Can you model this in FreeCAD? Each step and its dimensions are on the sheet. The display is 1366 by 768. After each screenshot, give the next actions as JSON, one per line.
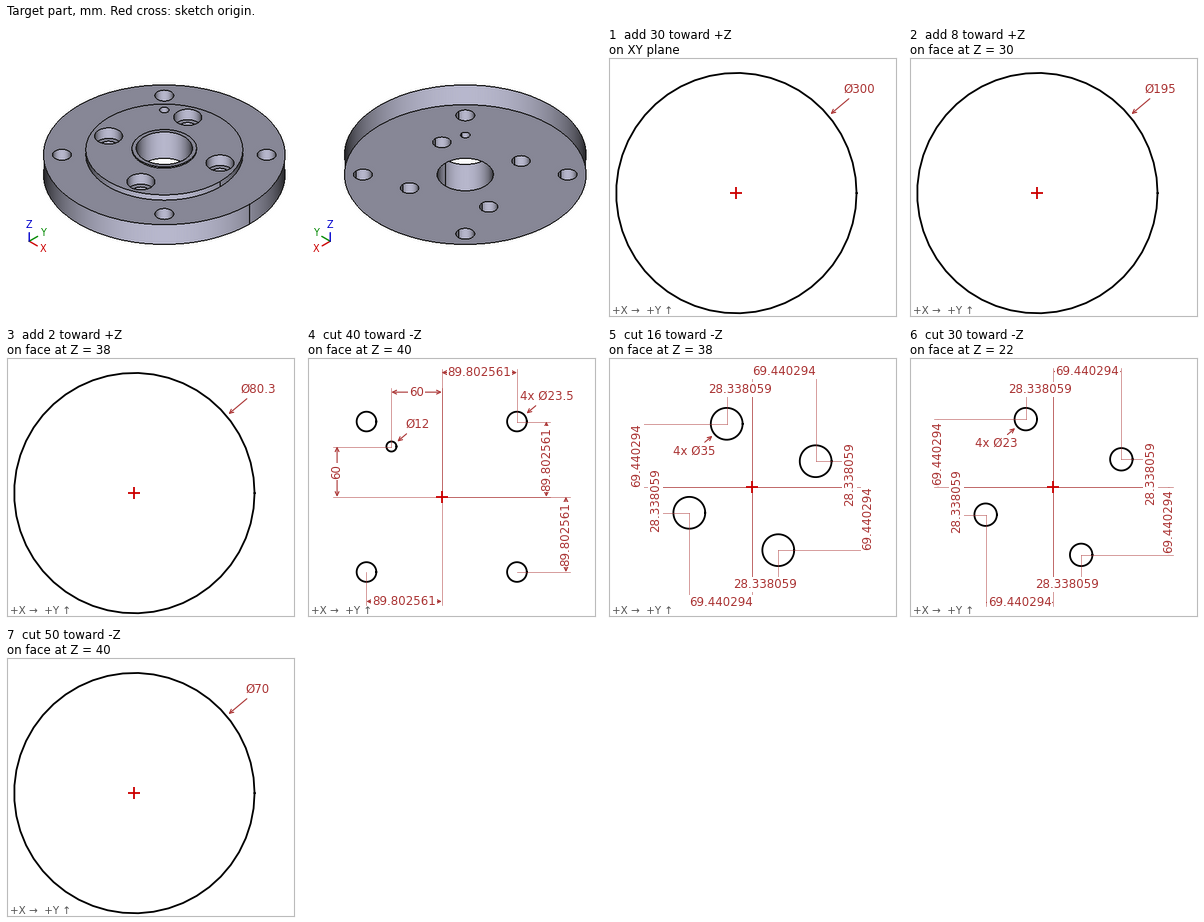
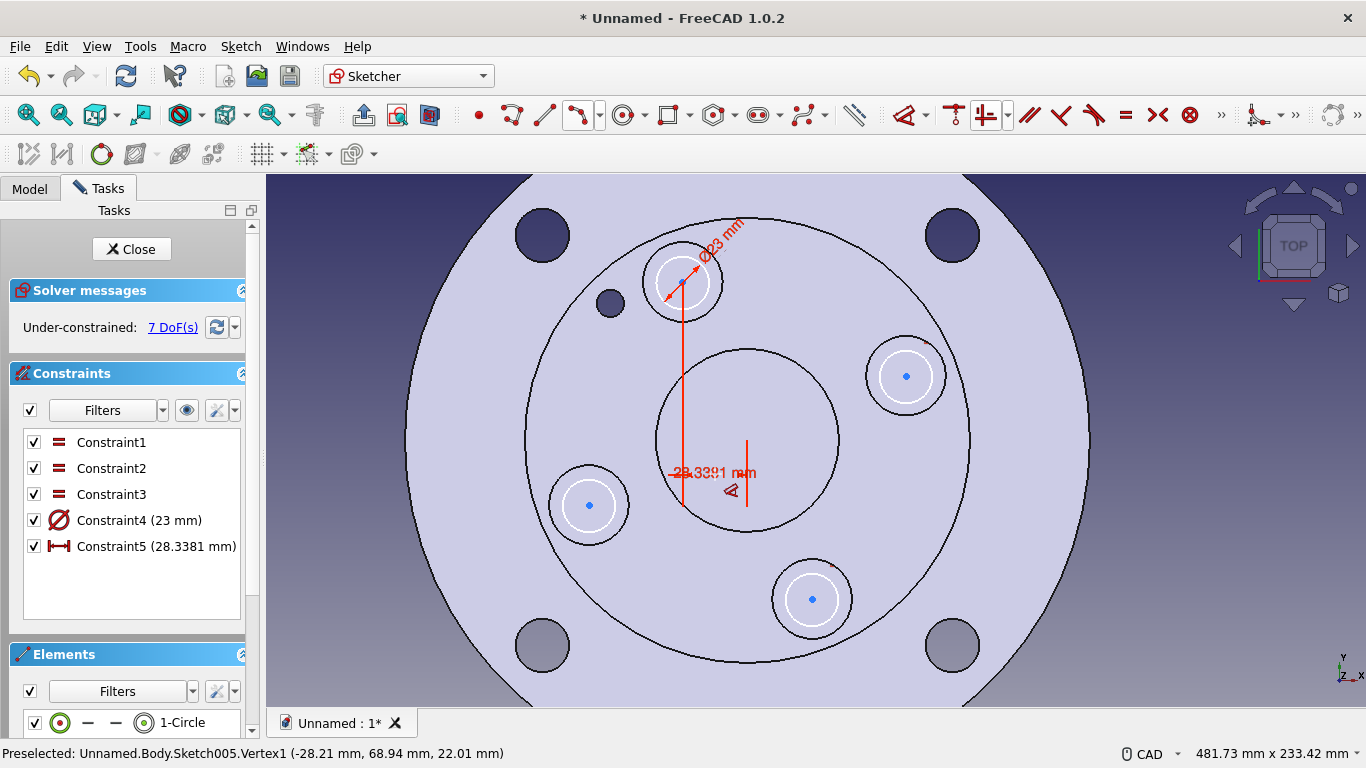
{"action": "left_click", "coordinate": [683, 283]}
{"action": "left_click", "coordinate": [649, 362]}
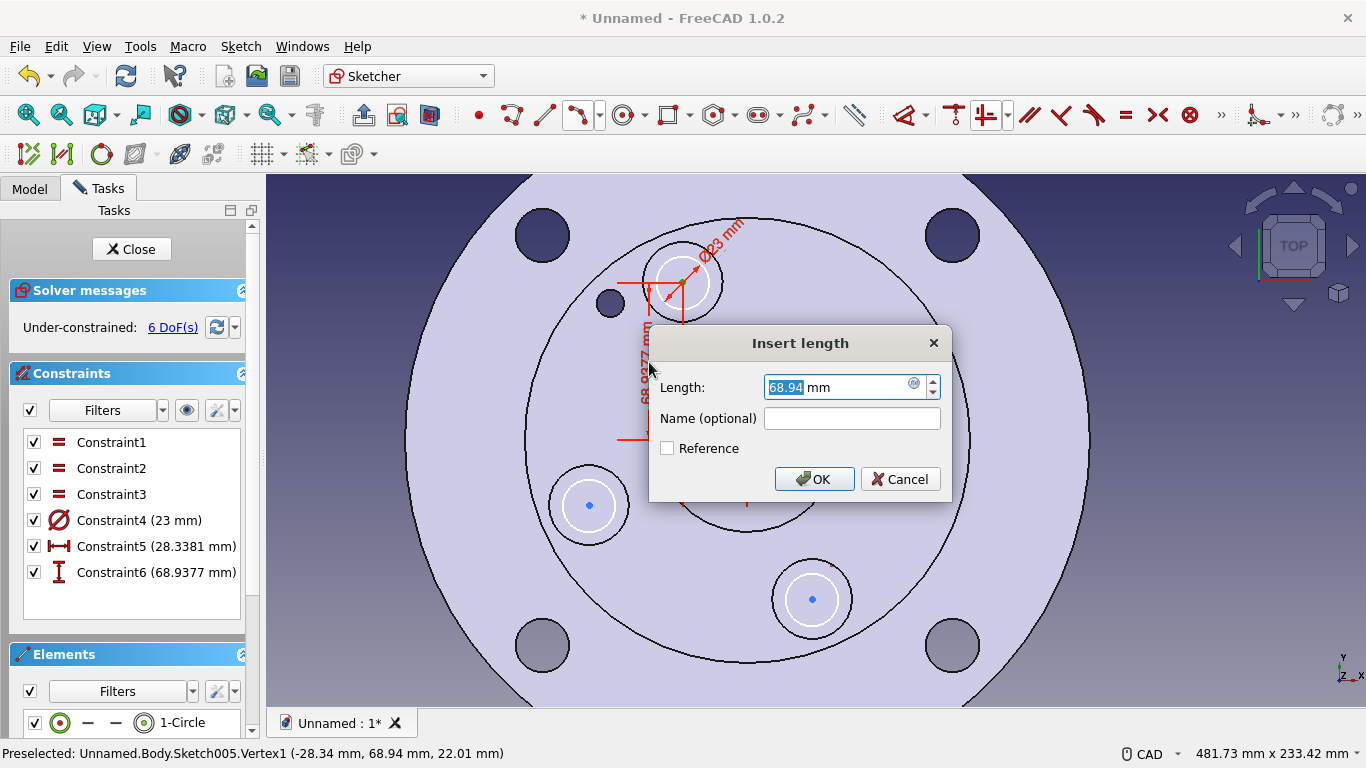
{"action": "type", "text": "69.440294"}
{"action": "key", "text": "Return"}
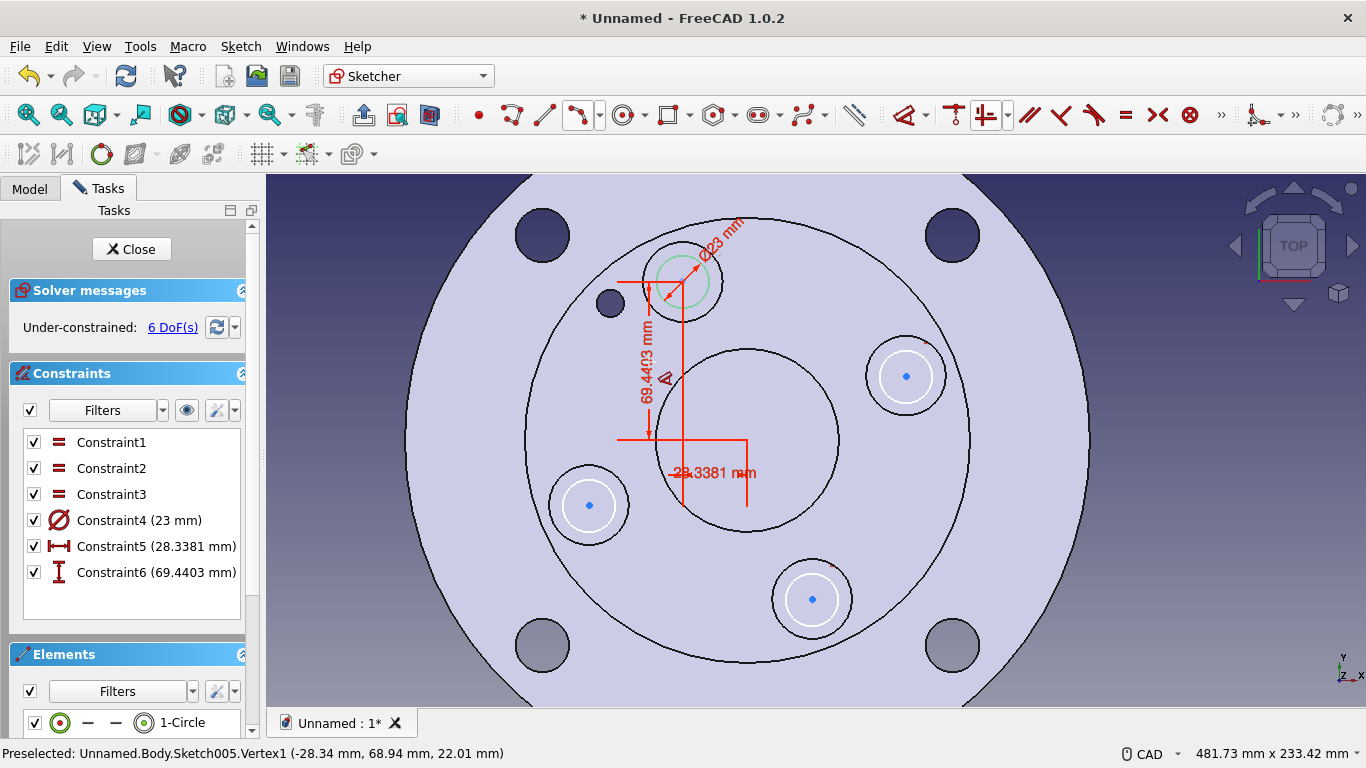
{"action": "left_click", "coordinate": [906, 377]}
{"action": "left_click", "coordinate": [827, 343]}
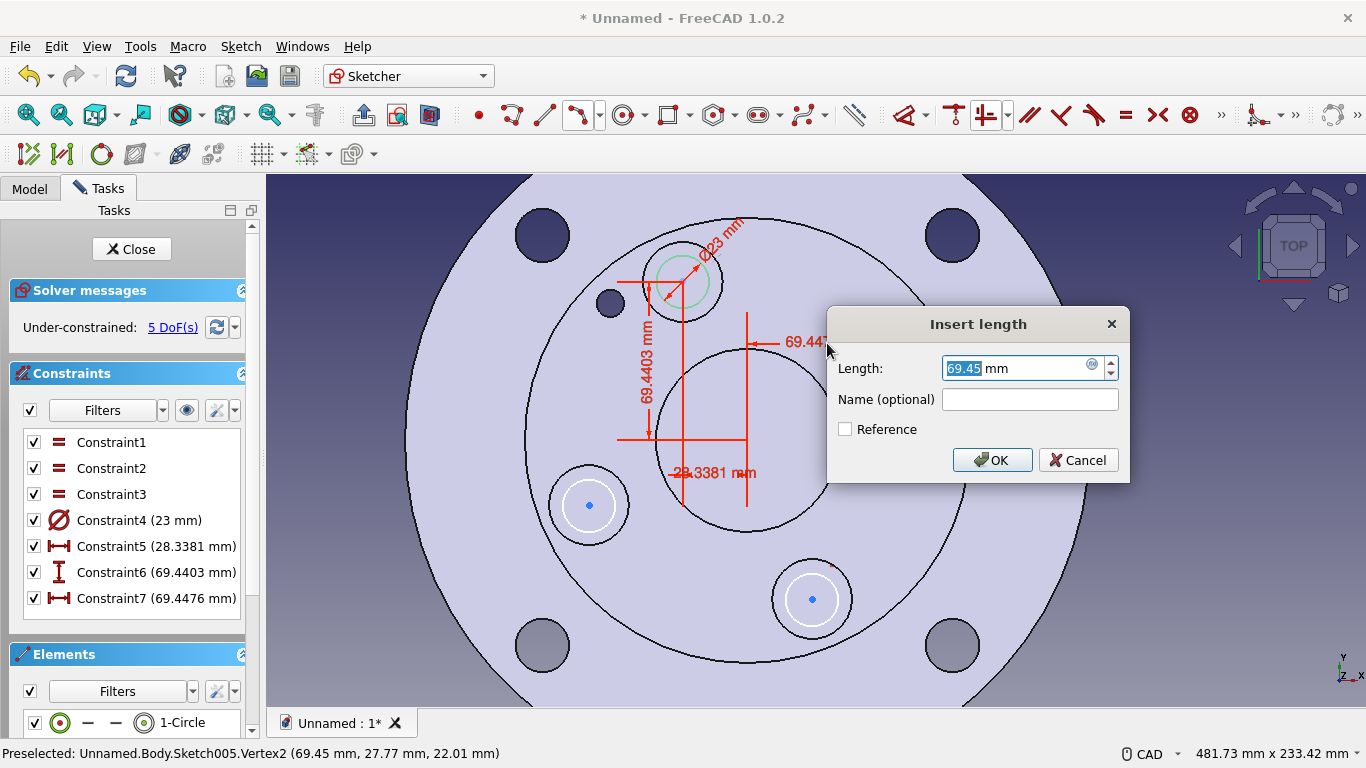
{"action": "type", "text": "69.440294"}
{"action": "key", "text": "Return"}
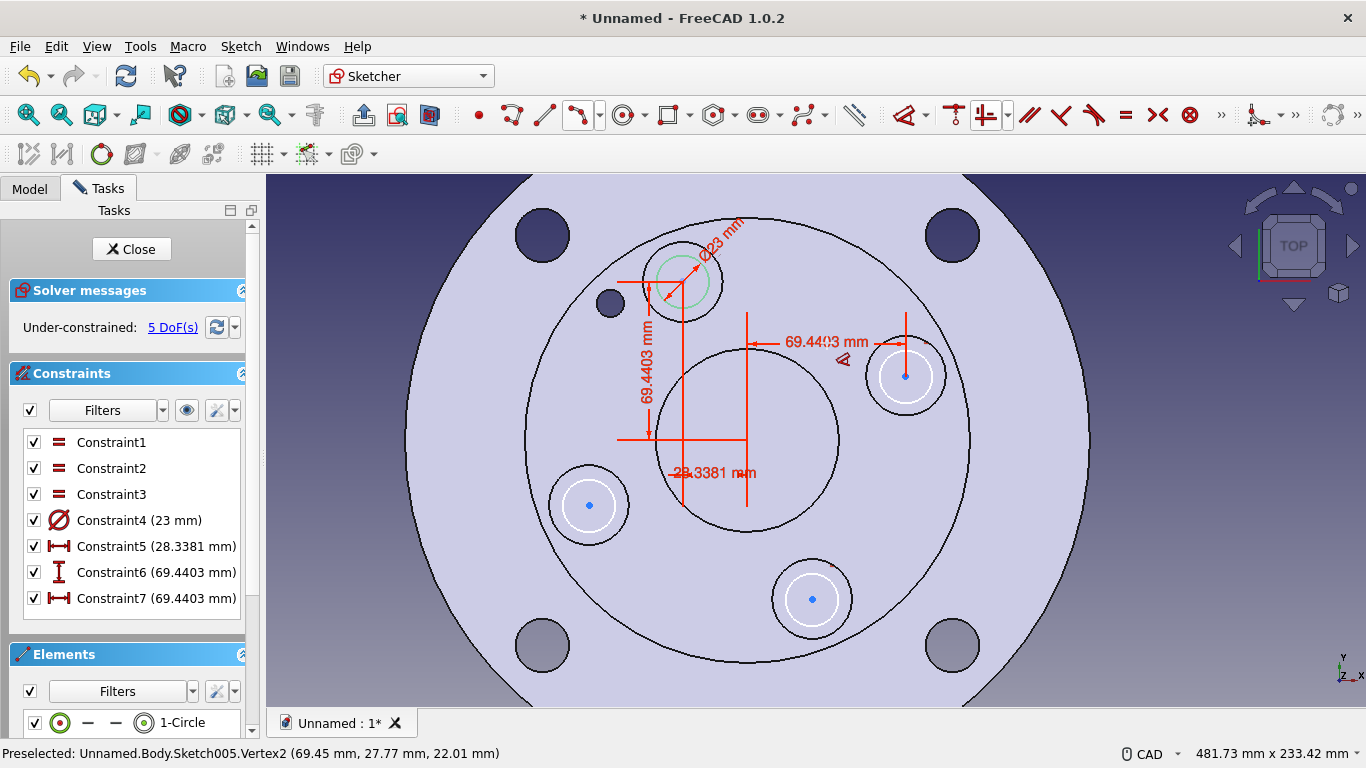
{"action": "left_click", "coordinate": [906, 377]}
{"action": "left_click", "coordinate": [940, 409]}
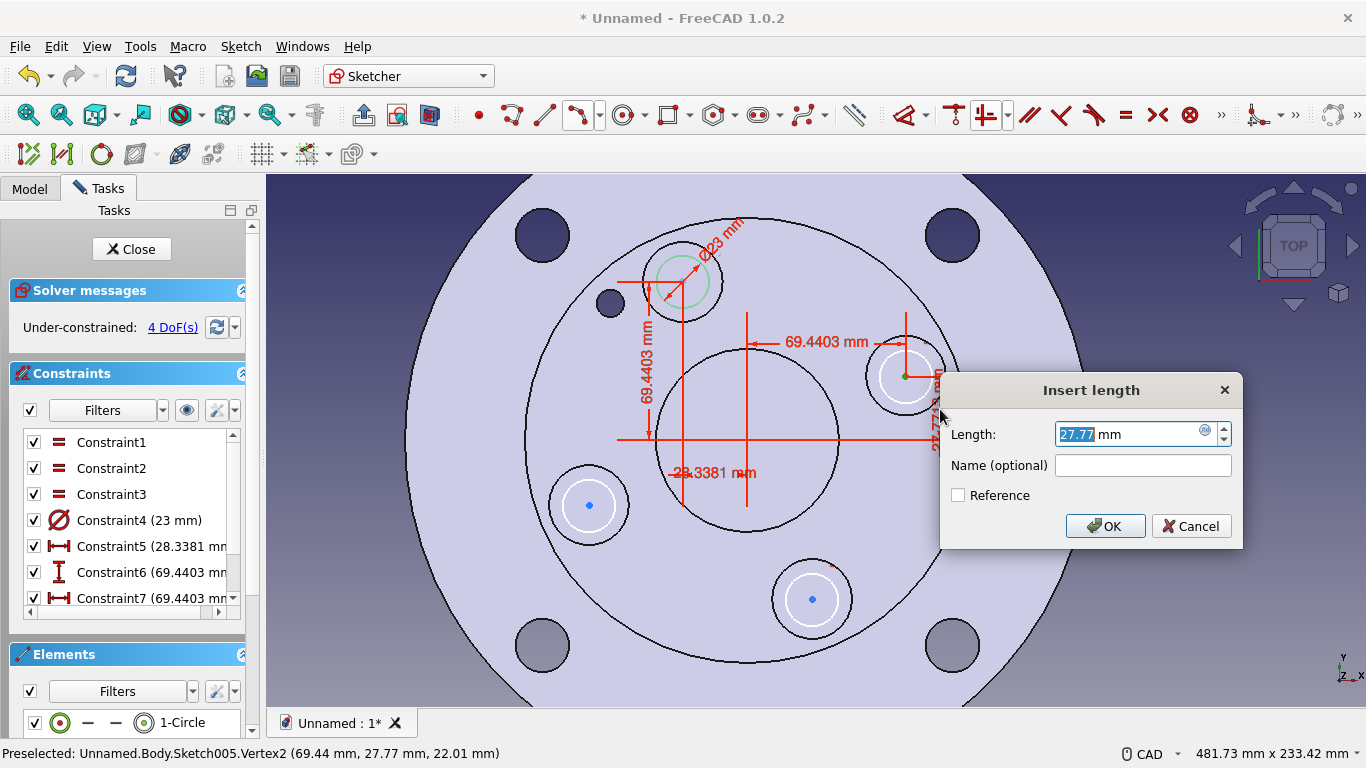
{"action": "type", "text": "28.338059"}
{"action": "key", "text": "Return"}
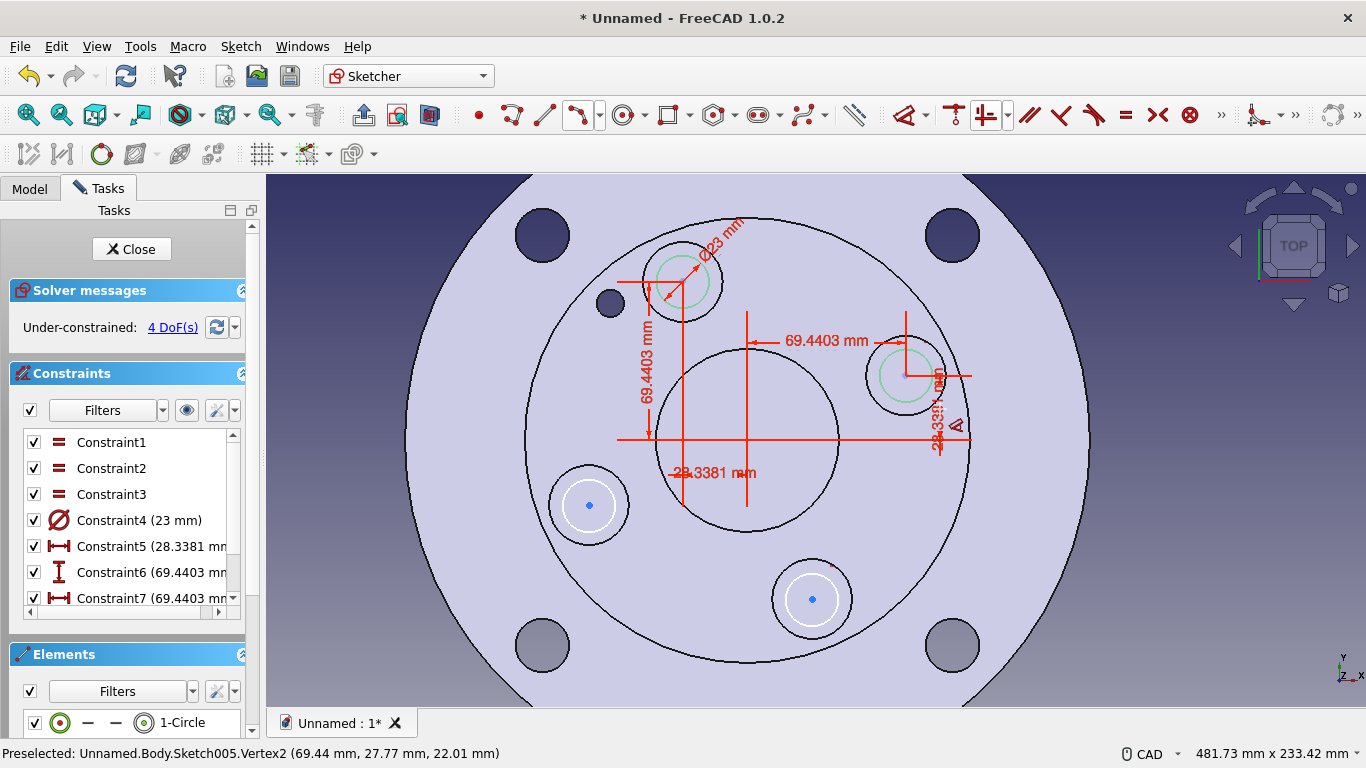
{"action": "left_click", "coordinate": [812, 600]}
{"action": "left_click", "coordinate": [780, 634]}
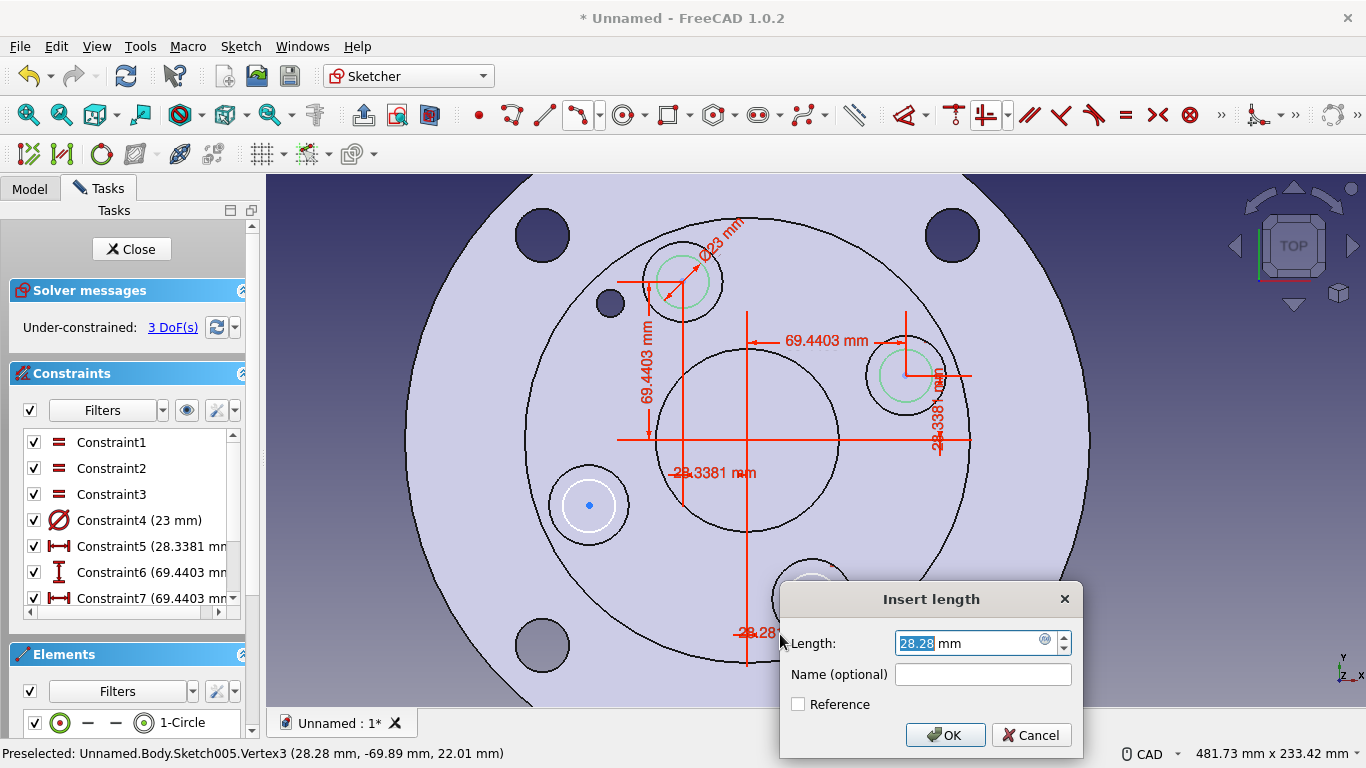
{"action": "type", "text": "28.338059"}
{"action": "key", "text": "Return"}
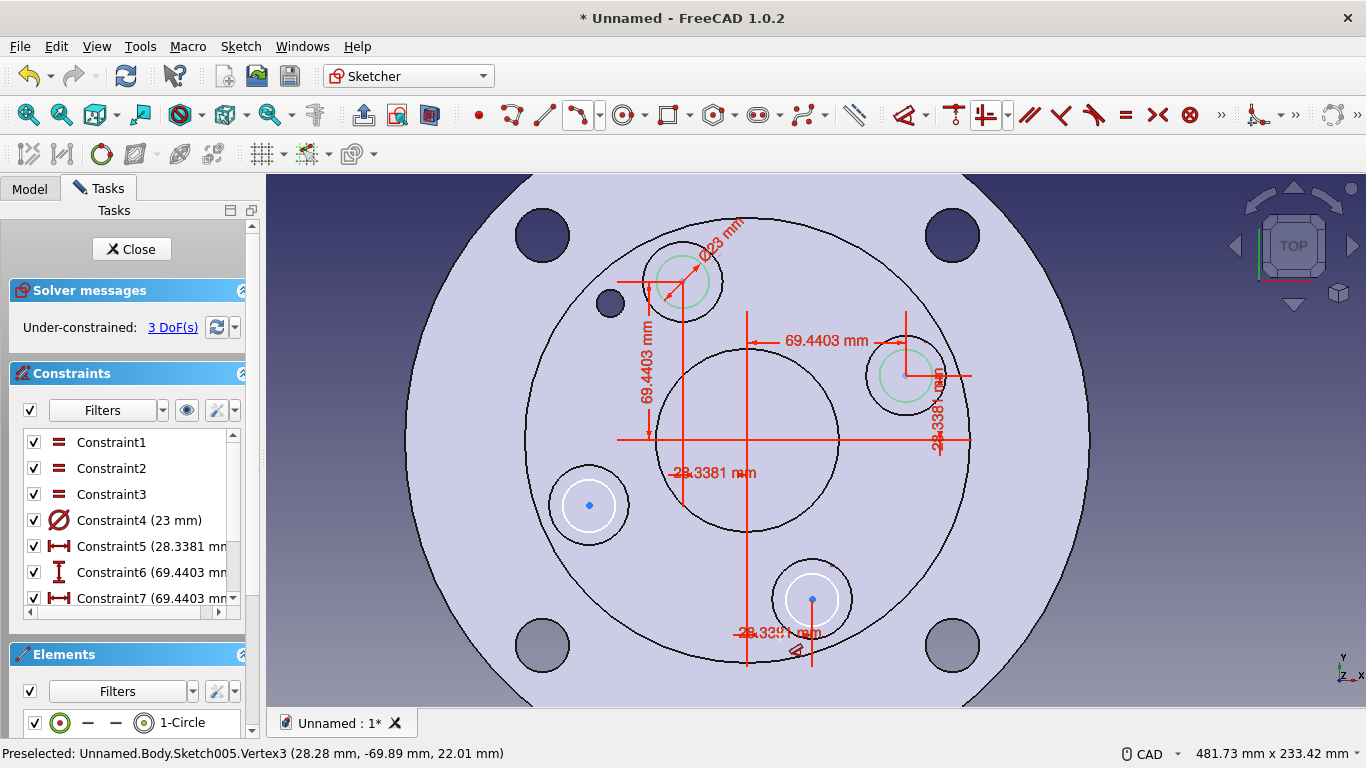
{"action": "left_click", "coordinate": [812, 600]}
{"action": "left_click", "coordinate": [846, 520]}